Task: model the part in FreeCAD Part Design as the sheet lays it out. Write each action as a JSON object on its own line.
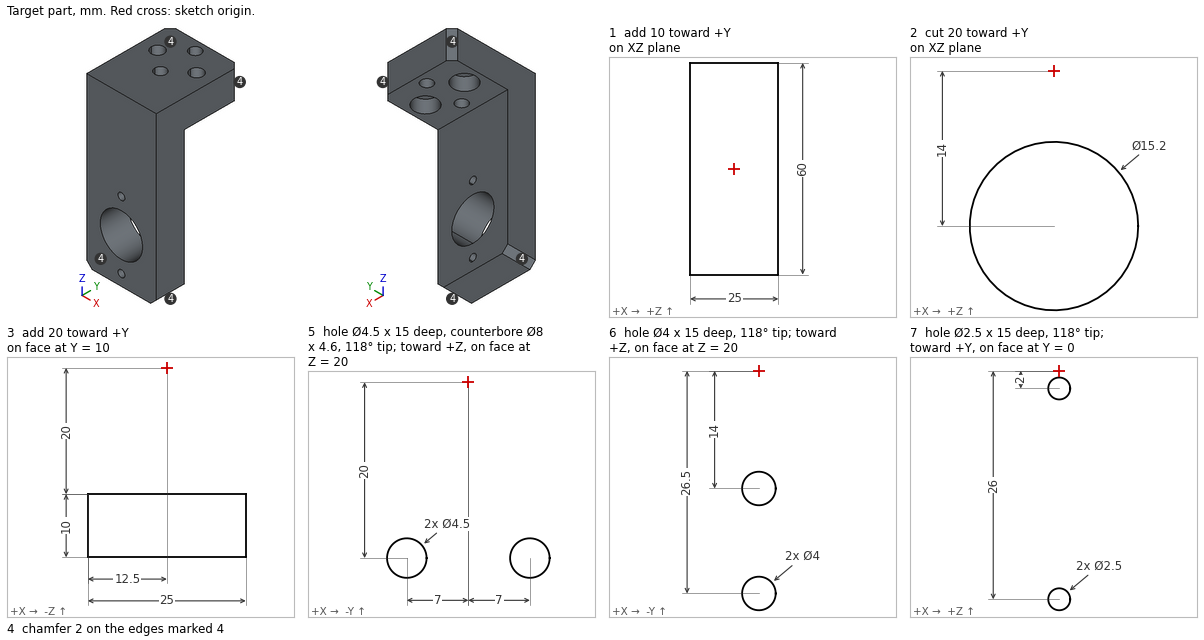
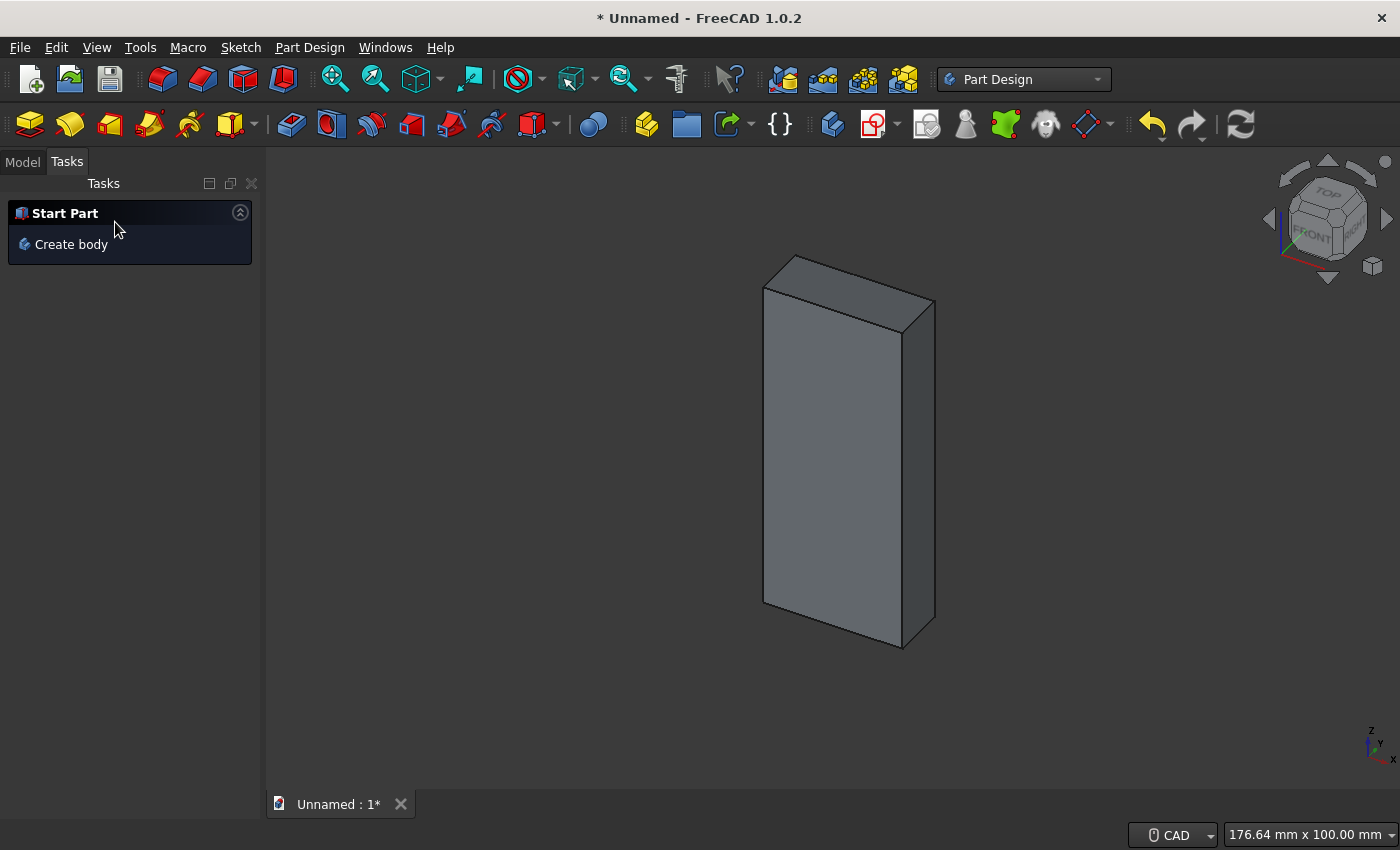
{"action": "left_click", "coordinate": [874, 124]}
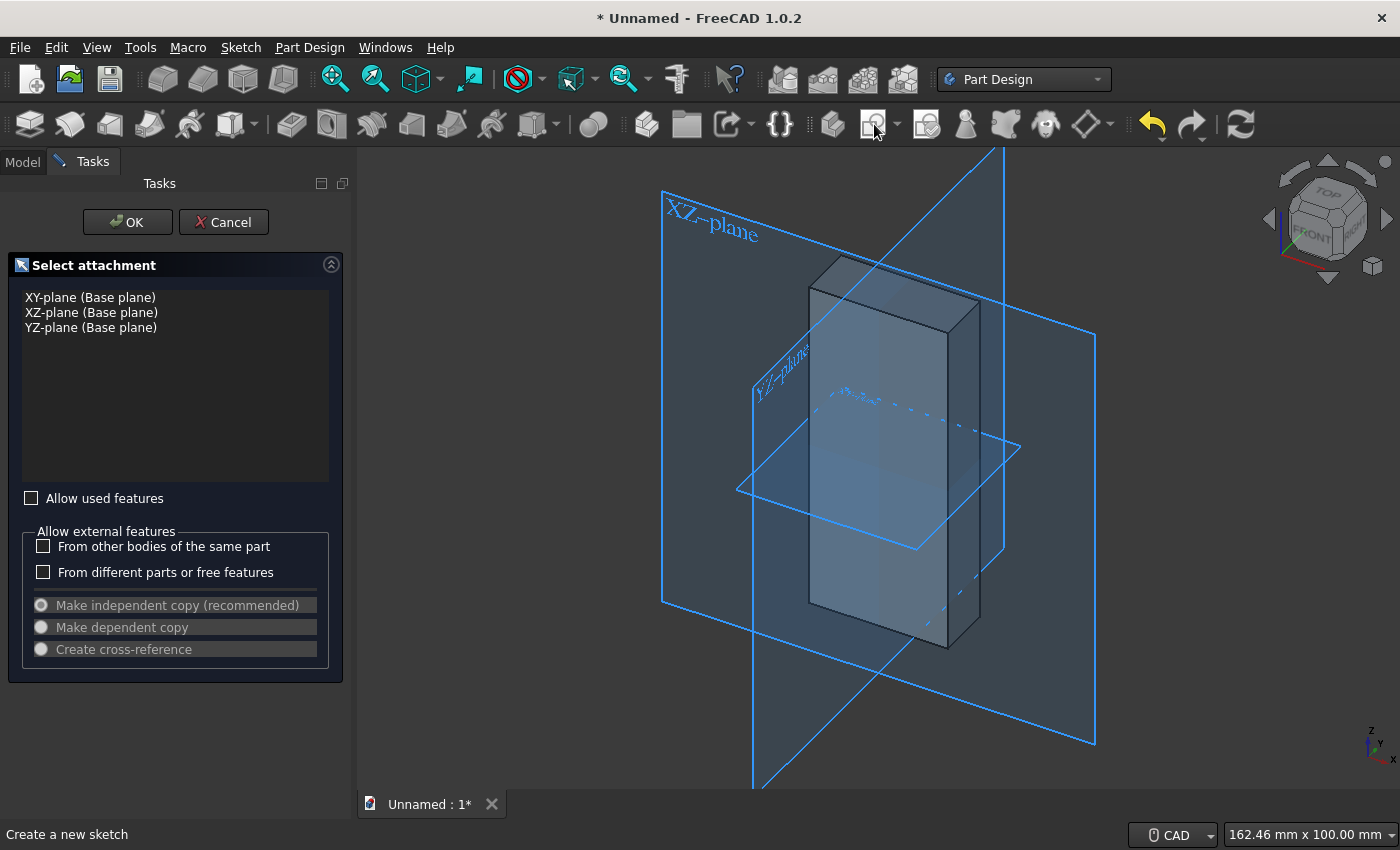
{"action": "left_click", "coordinate": [82, 312]}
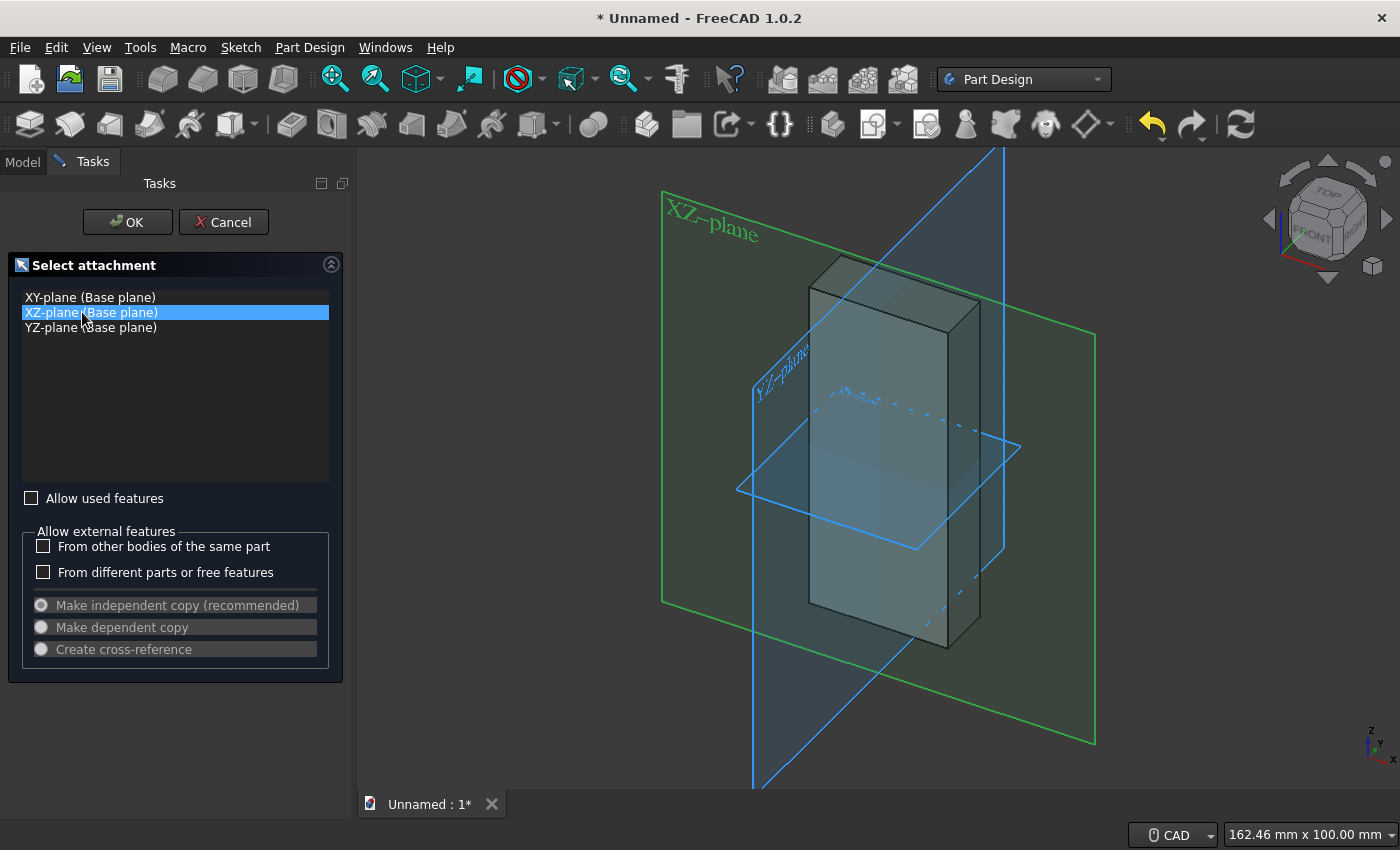
{"action": "left_click", "coordinate": [128, 222]}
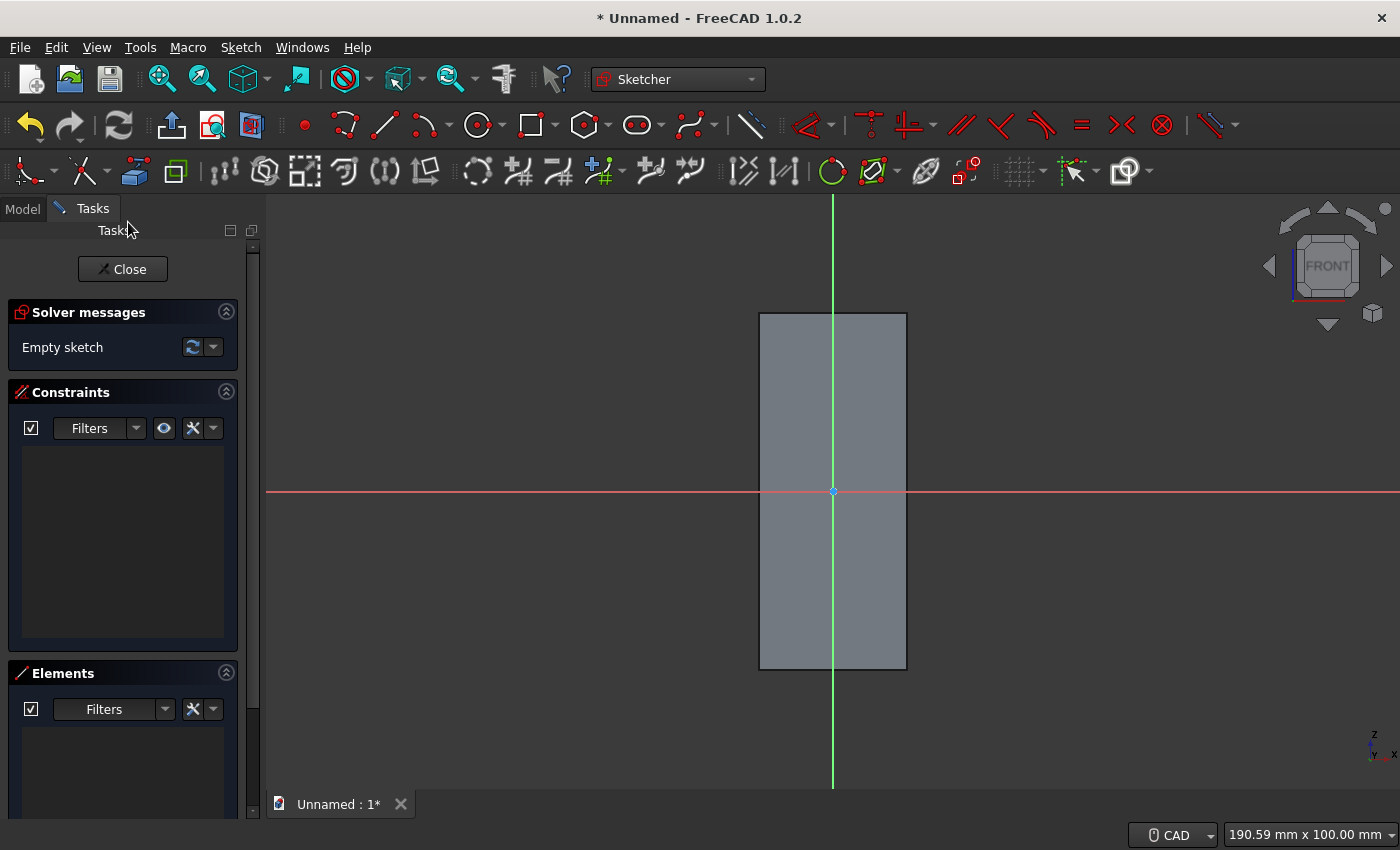
{"action": "scroll", "coordinate": [873, 593], "scroll_direction": "up", "scroll_amount": 5}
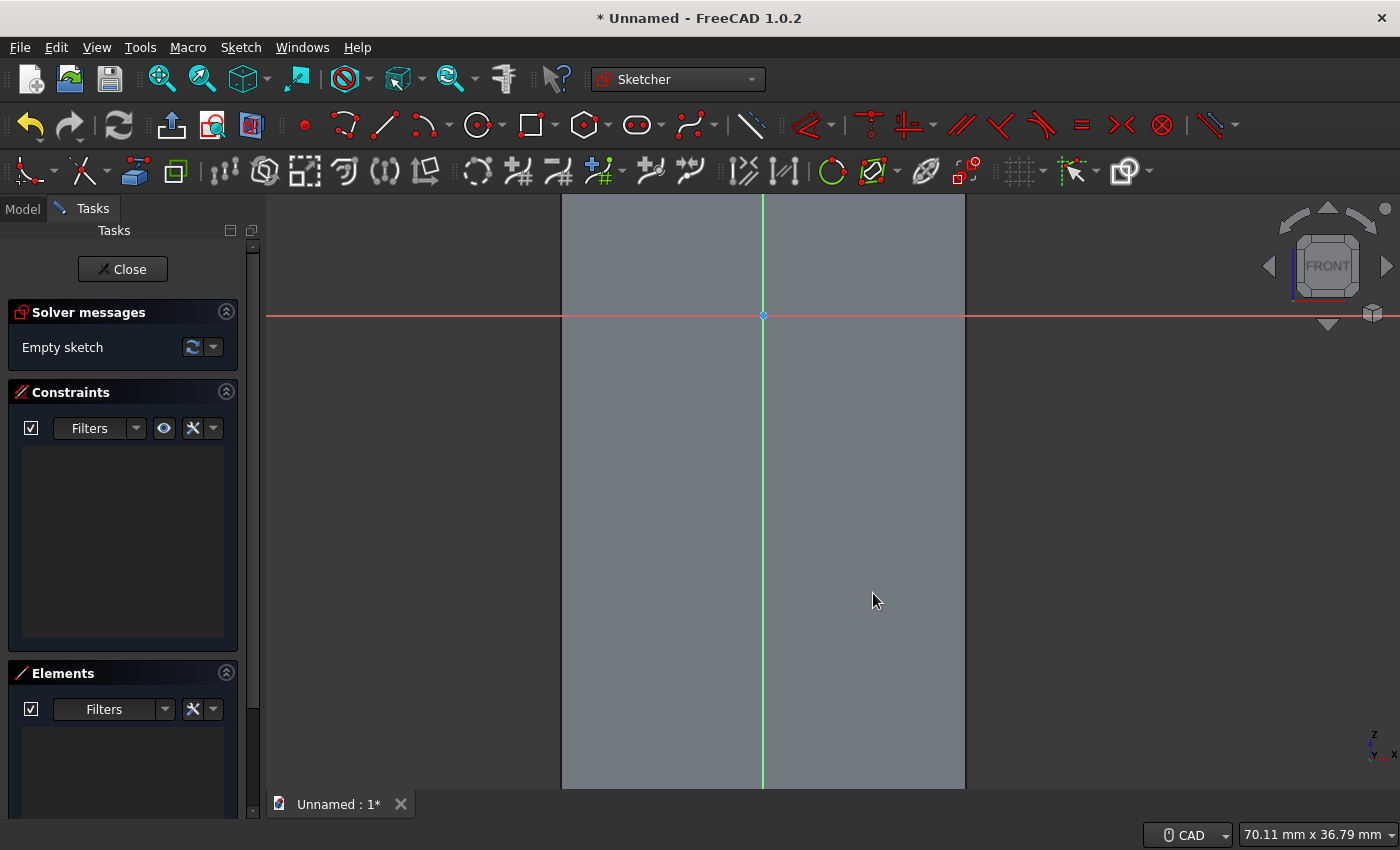
{"action": "left_click", "coordinate": [478, 126]}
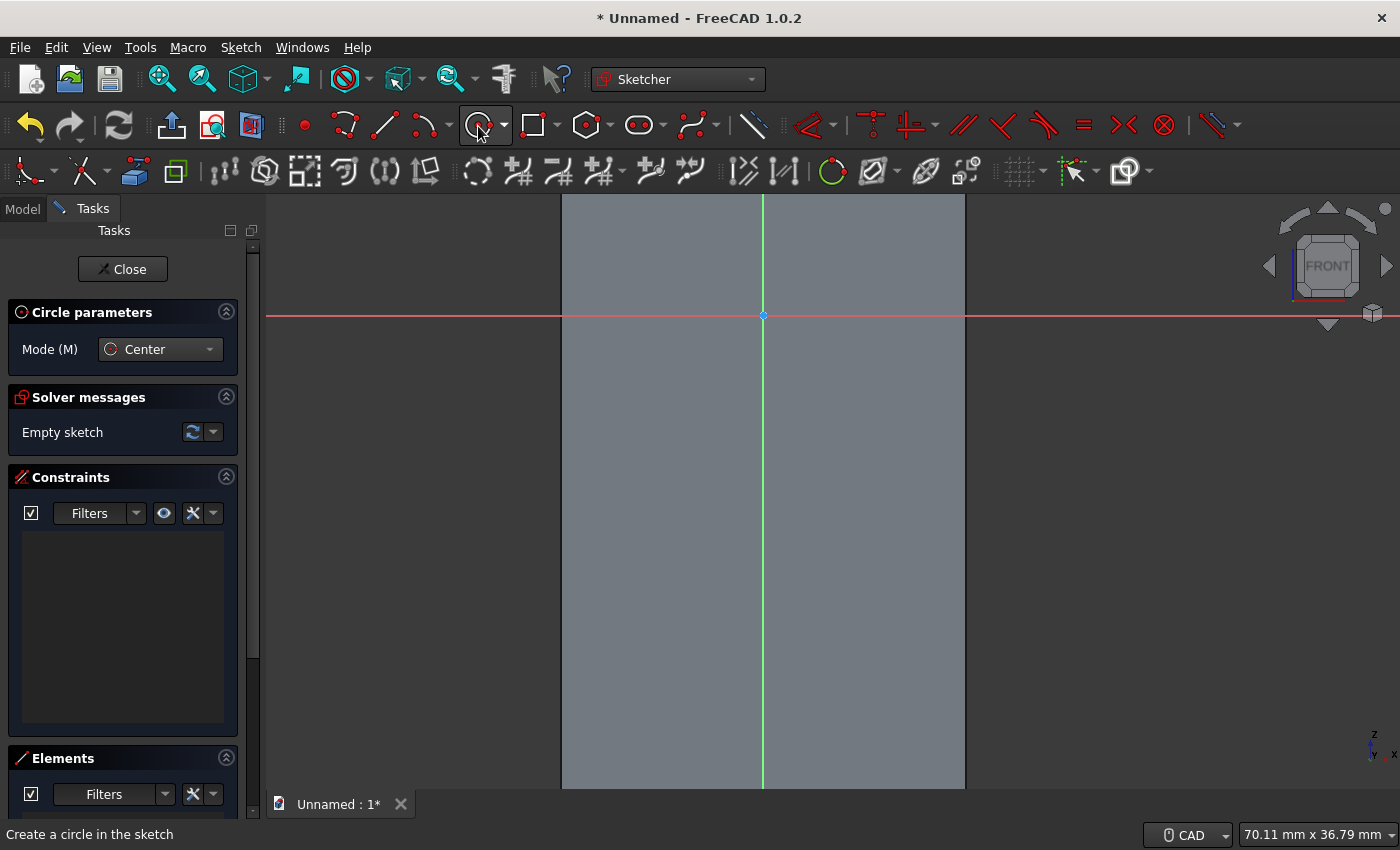
{"action": "left_click", "coordinate": [763, 542]}
{"action": "left_click", "coordinate": [850, 455]}
{"action": "key", "text": "Escape"}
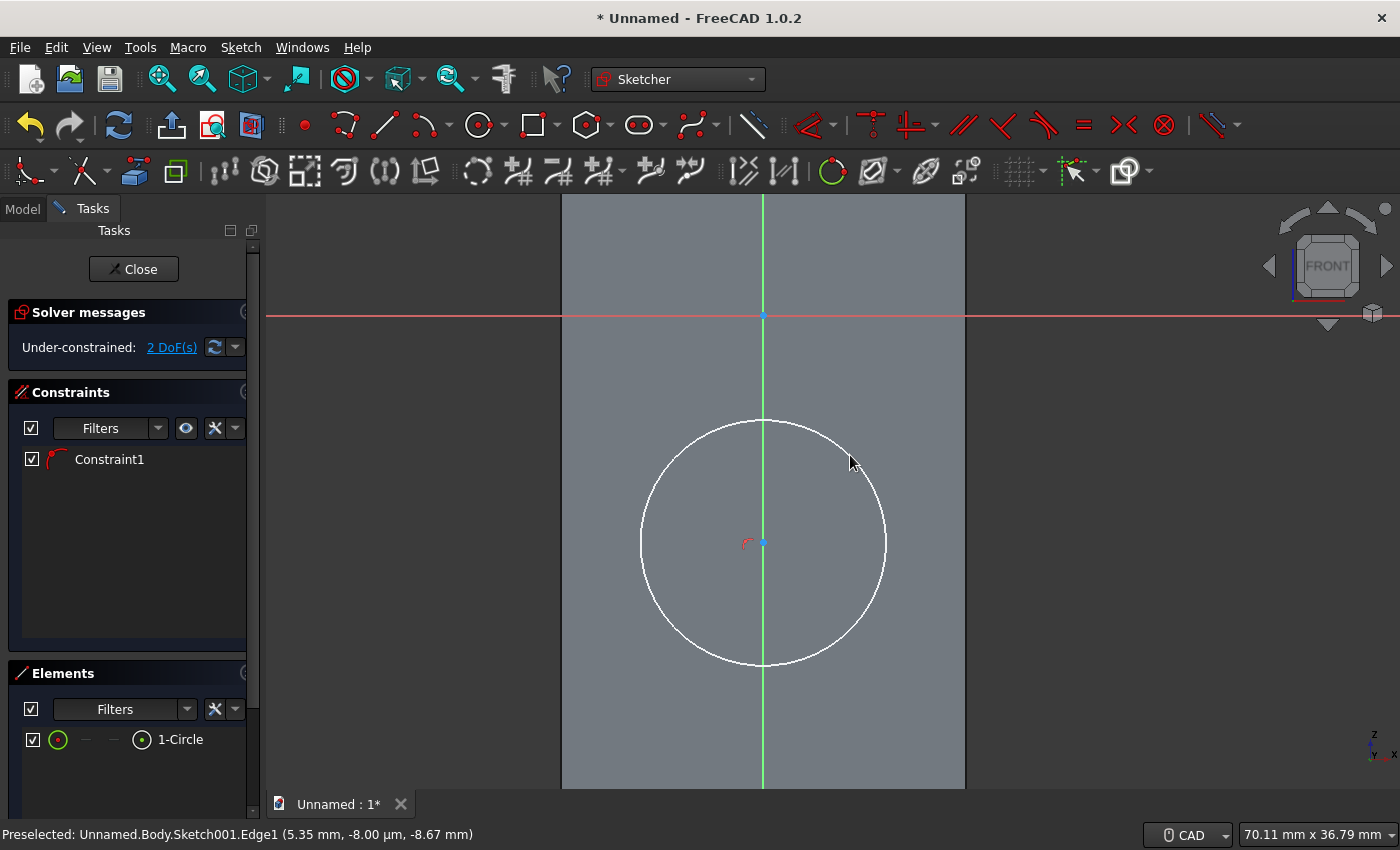
{"action": "left_click", "coordinate": [808, 126]}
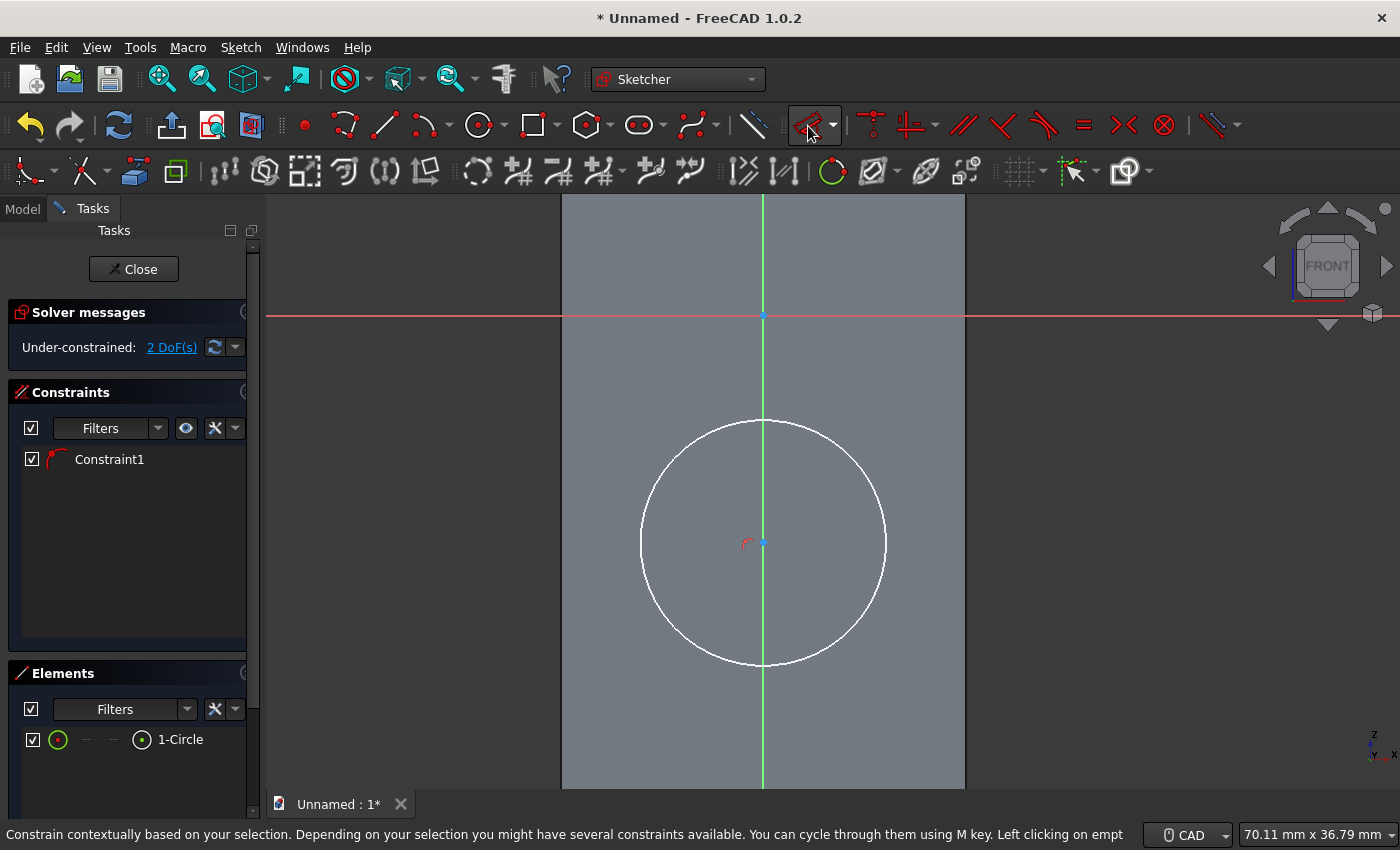
{"action": "left_click", "coordinate": [850, 456]}
{"action": "left_click", "coordinate": [873, 433]}